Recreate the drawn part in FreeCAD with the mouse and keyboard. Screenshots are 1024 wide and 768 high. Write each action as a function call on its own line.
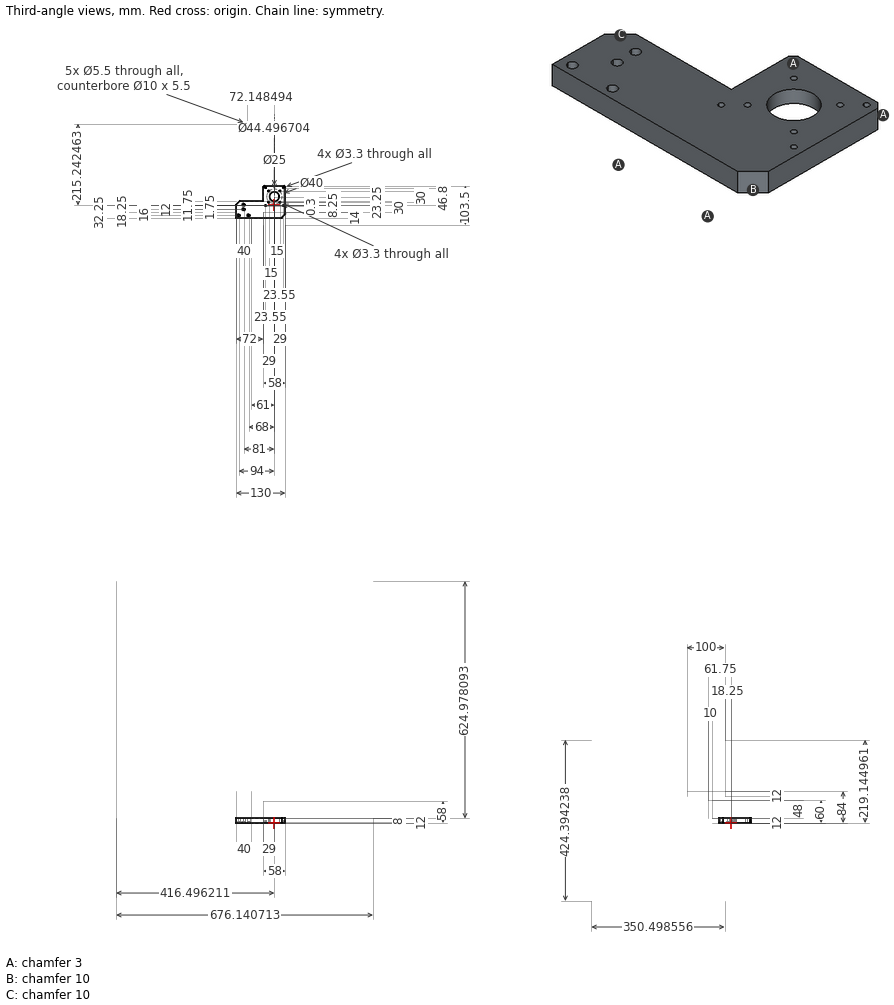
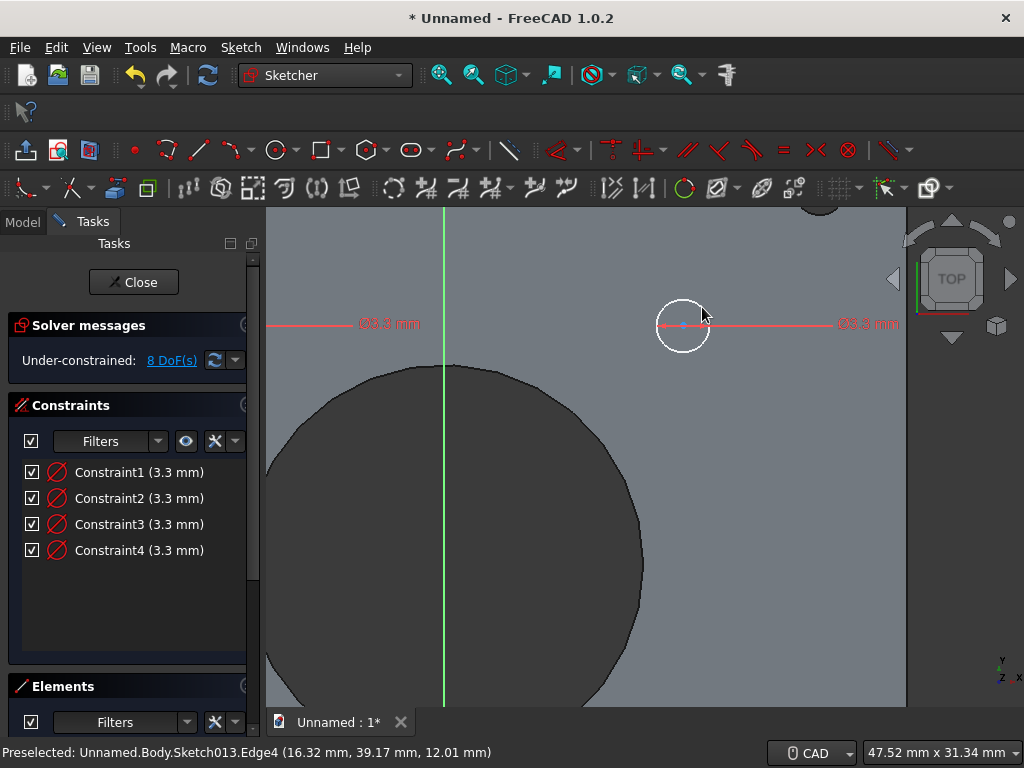
scroll(685, 326, down, 4)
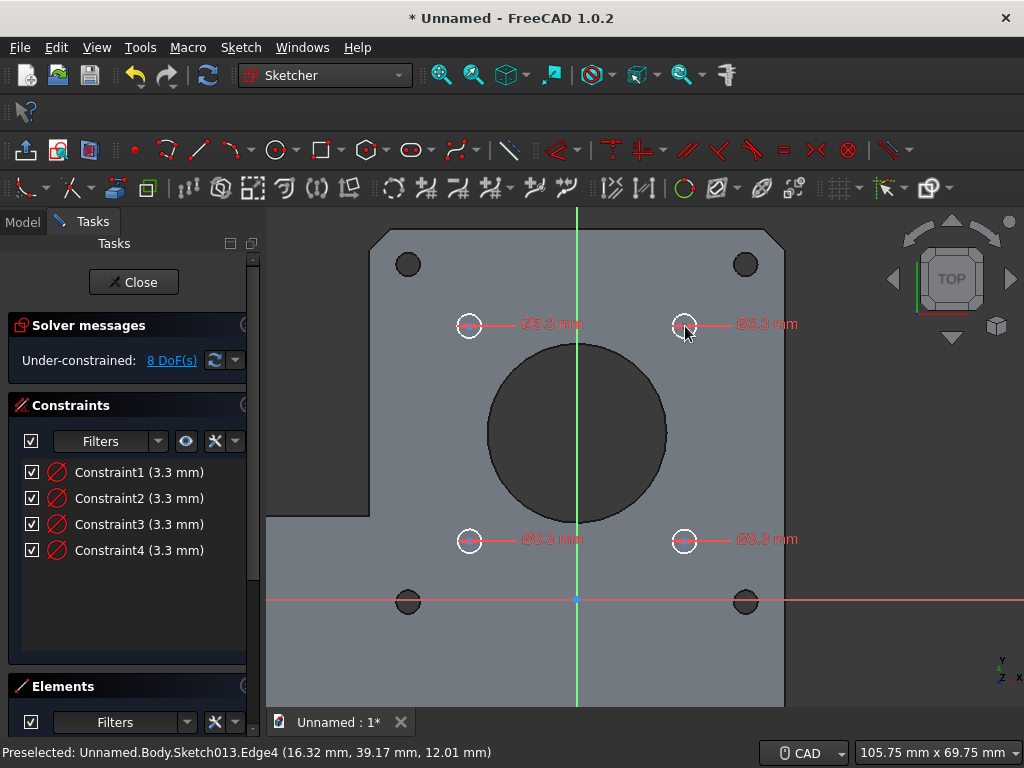
click(684, 541)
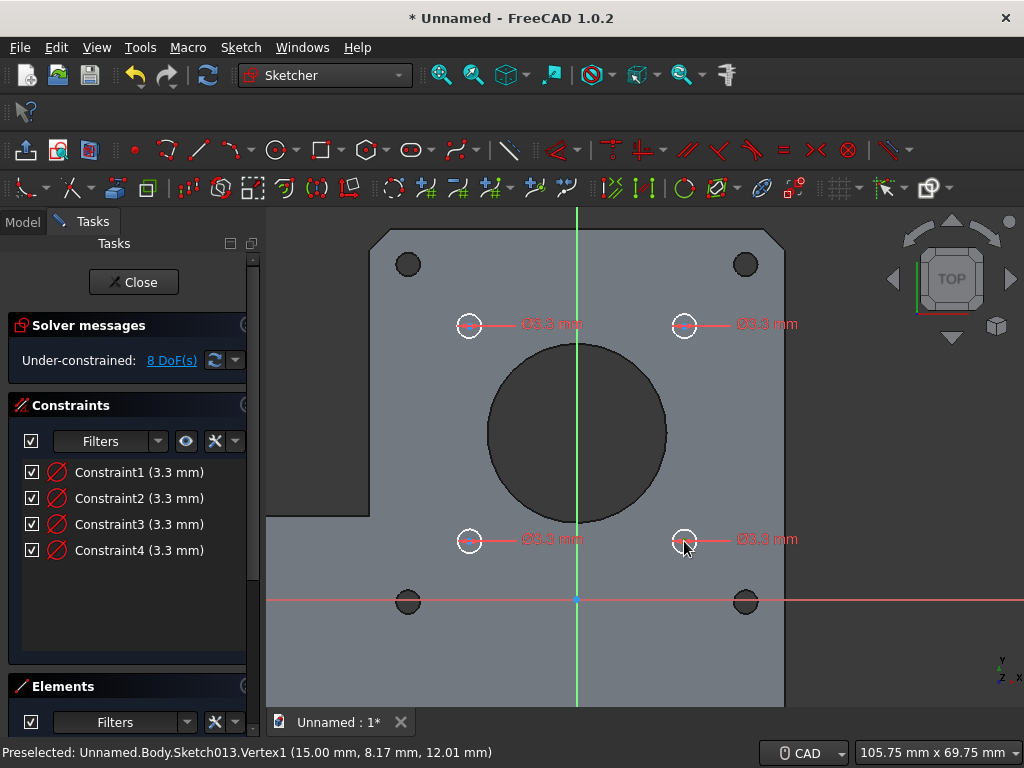
click(470, 541)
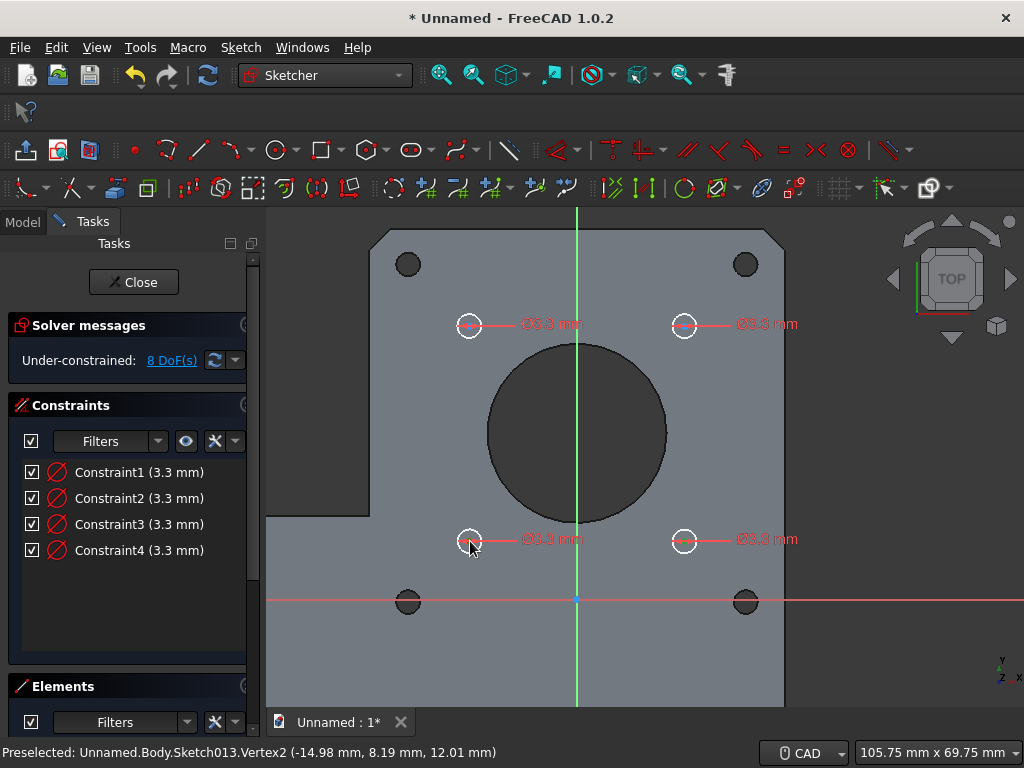
click(577, 647)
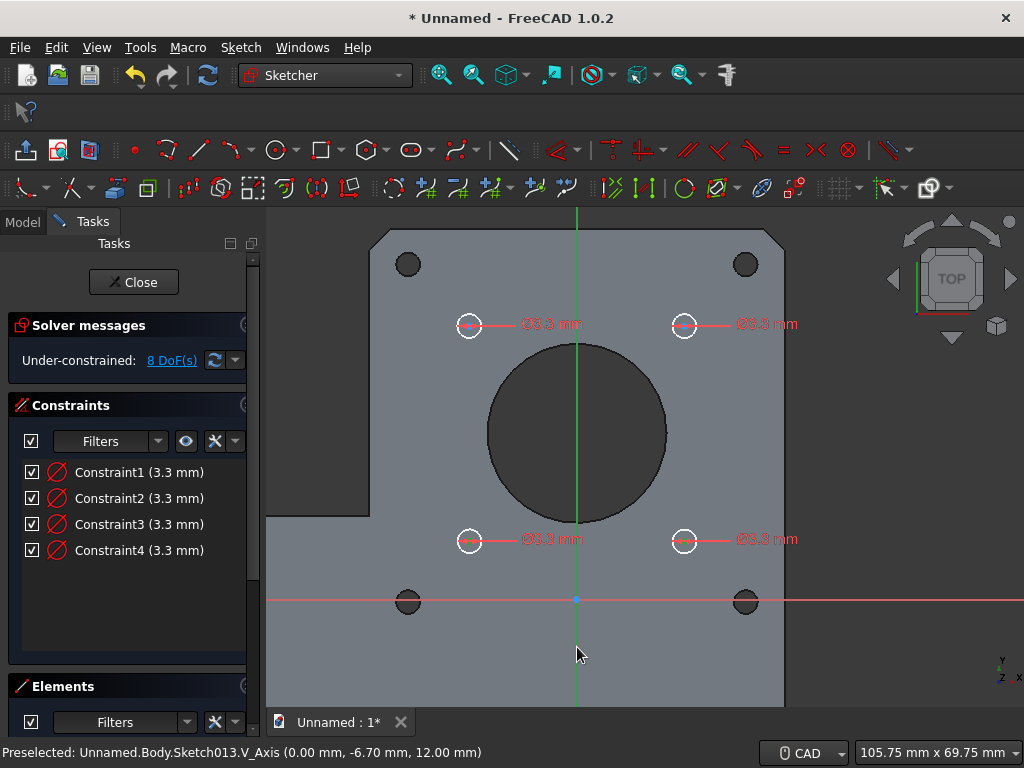
click(816, 150)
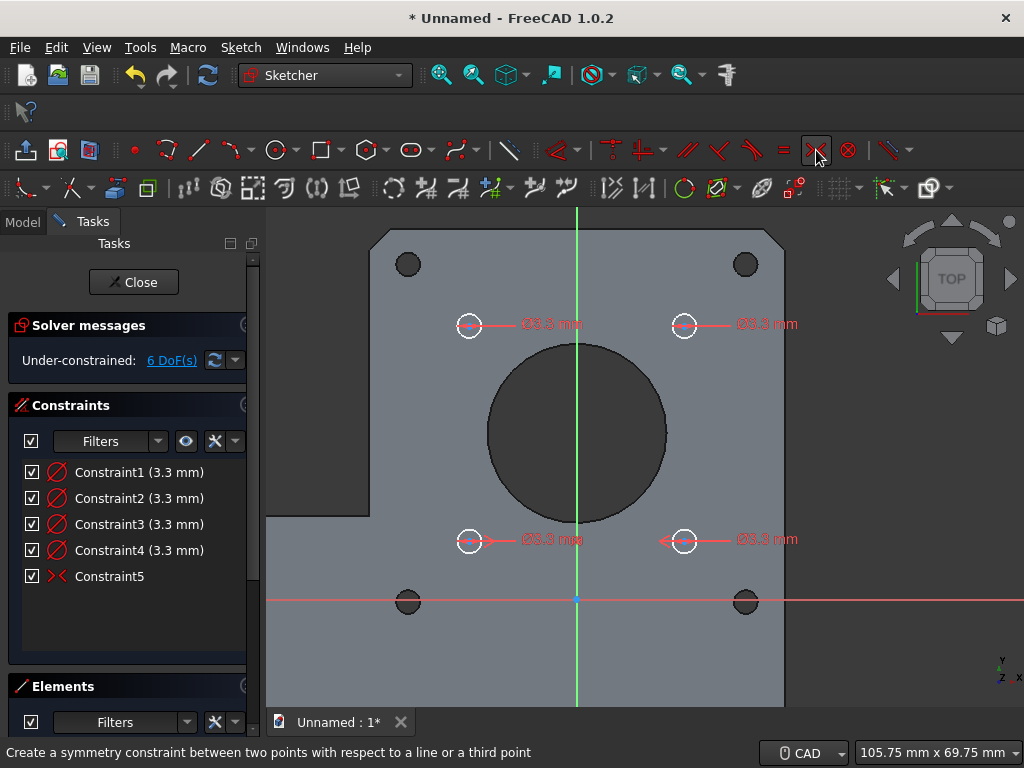
click(469, 326)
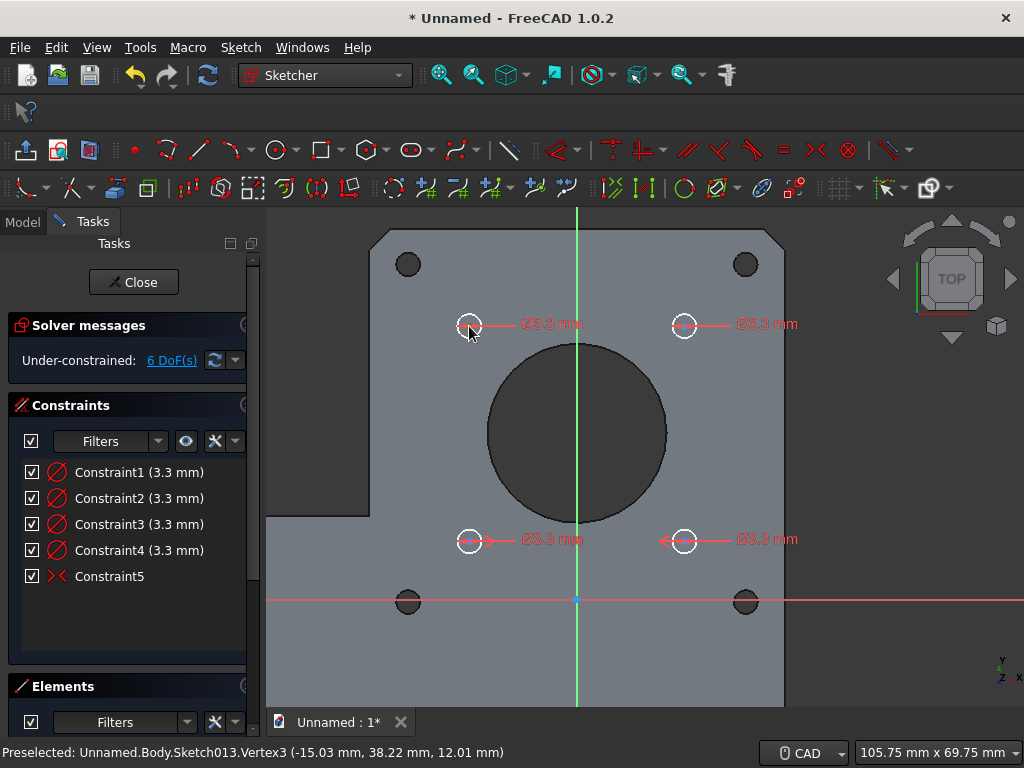
click(684, 326)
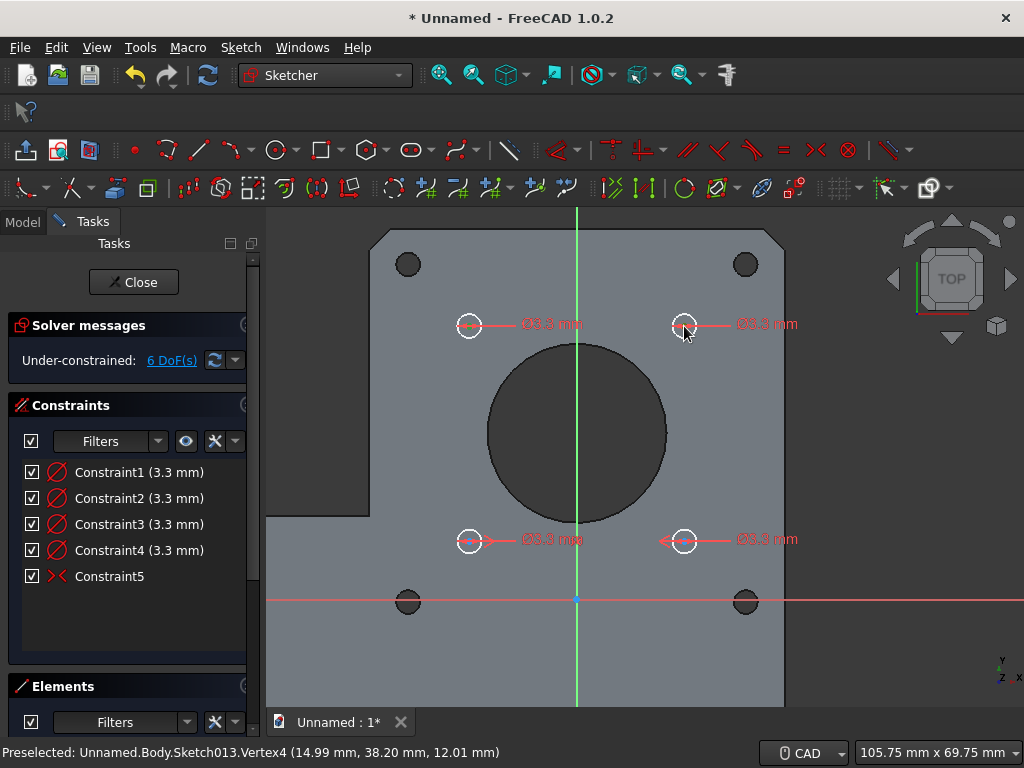
click(577, 647)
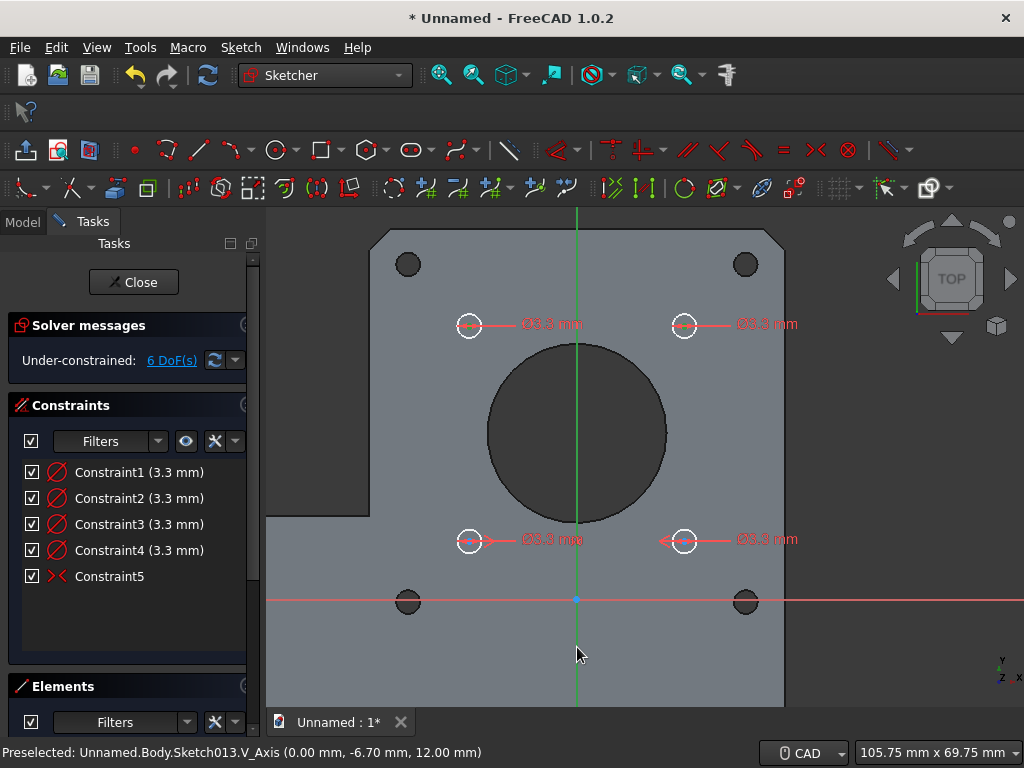
click(816, 150)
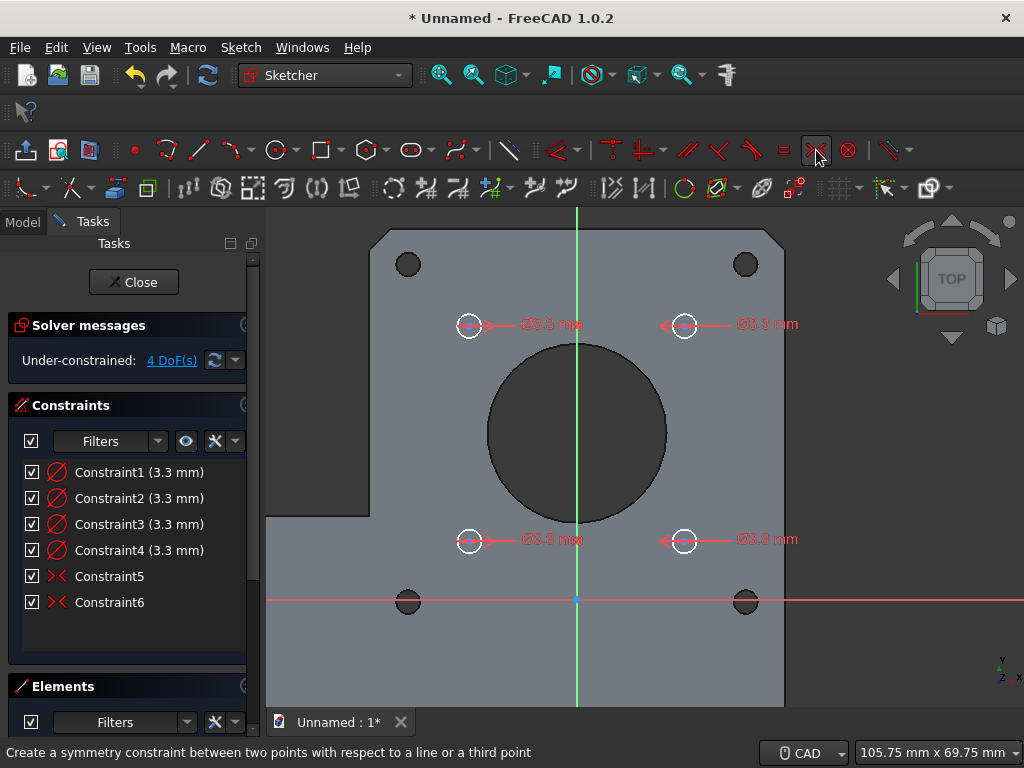
click(556, 150)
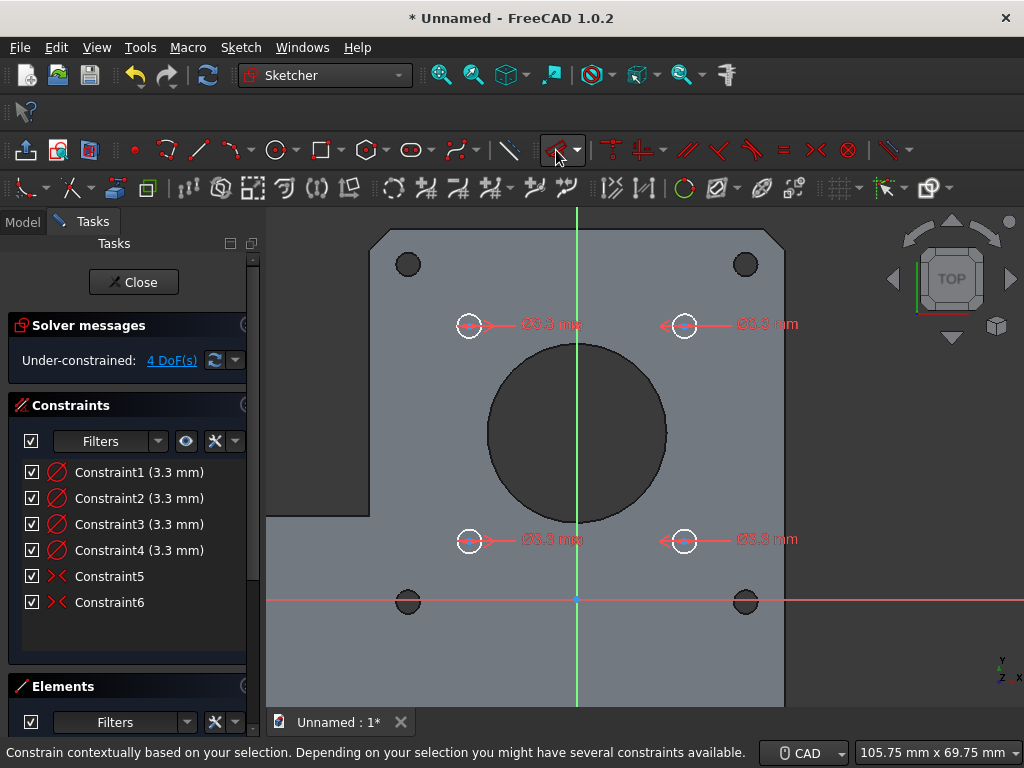
click(684, 541)
click(631, 634)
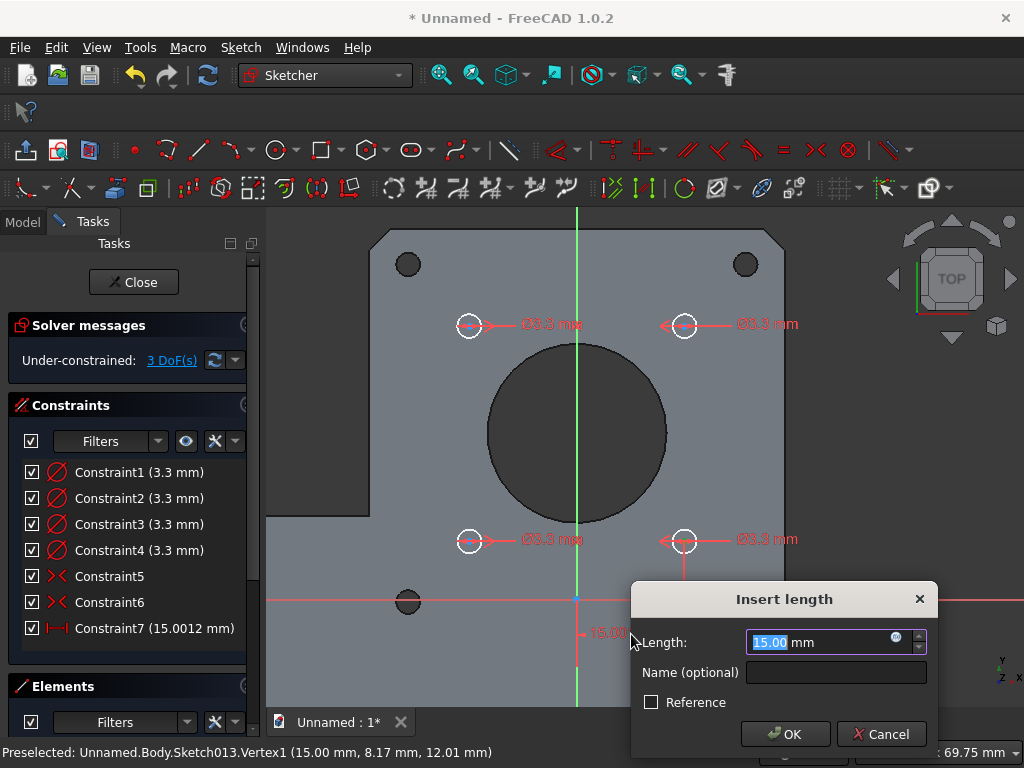
text(15)
key(Return)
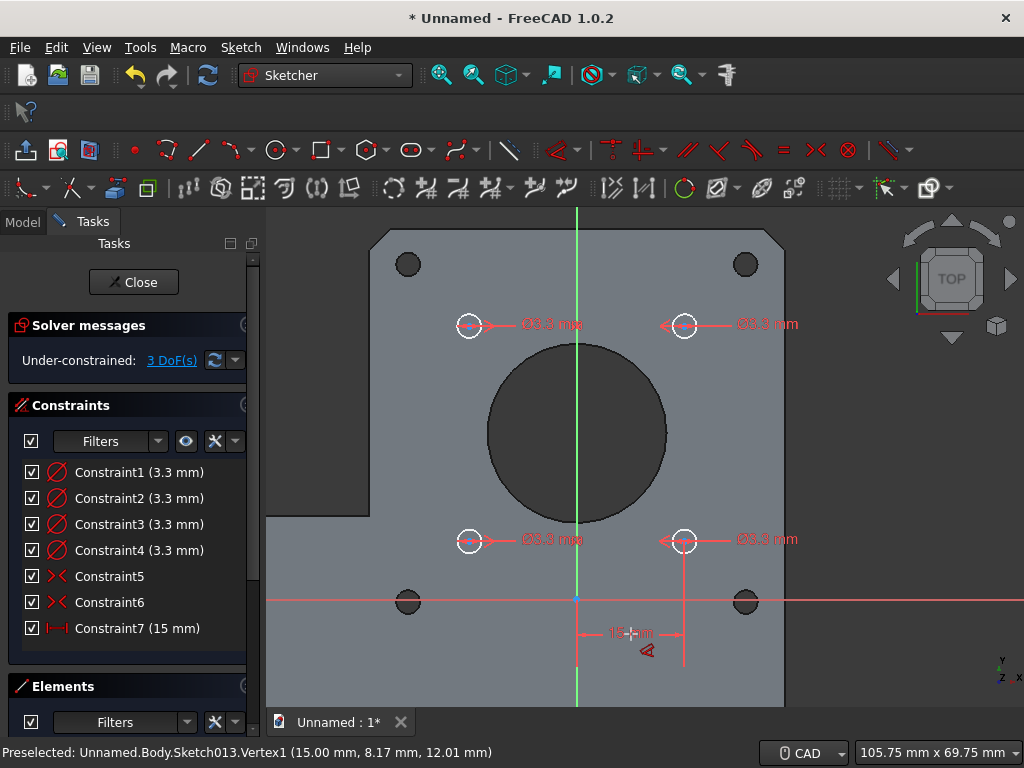
click(469, 326)
click(523, 634)